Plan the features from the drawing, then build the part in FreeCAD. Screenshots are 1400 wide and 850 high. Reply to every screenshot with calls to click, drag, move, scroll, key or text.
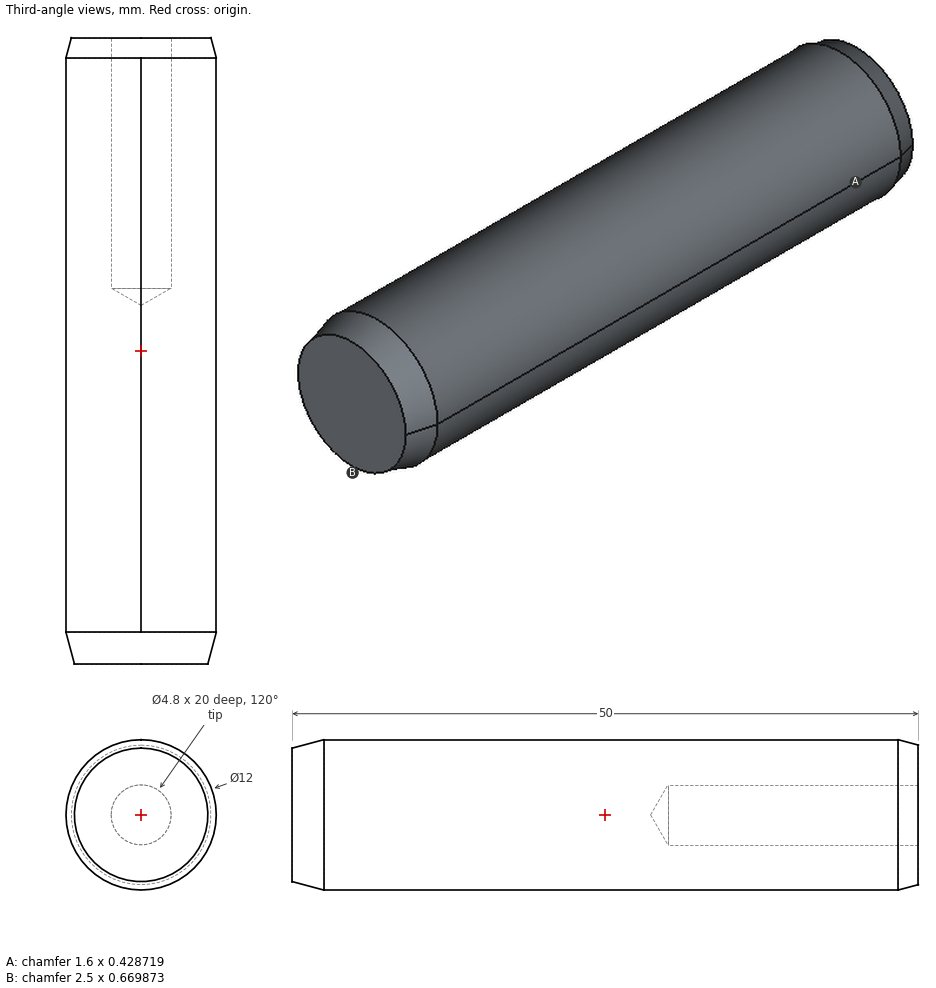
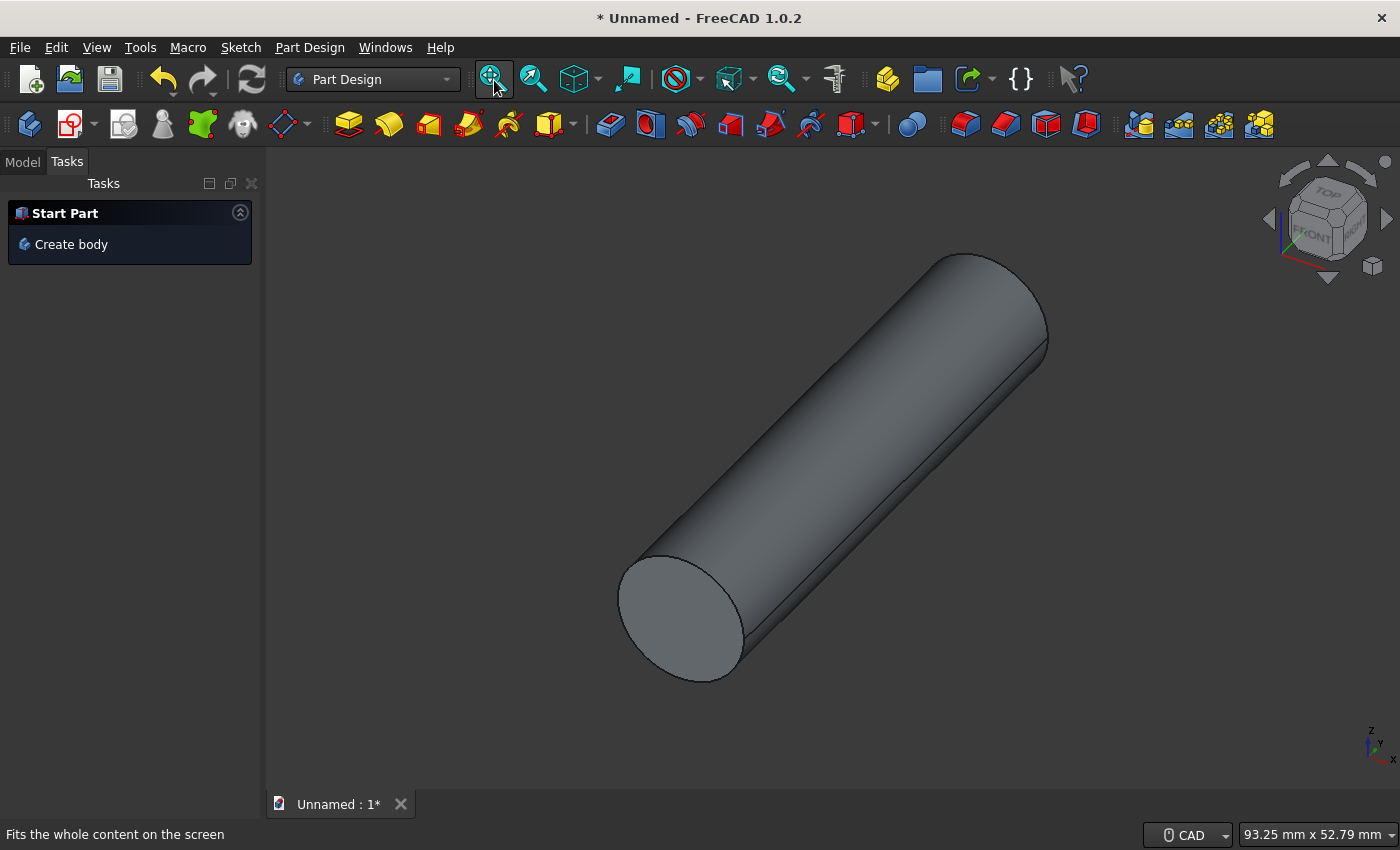
key(4)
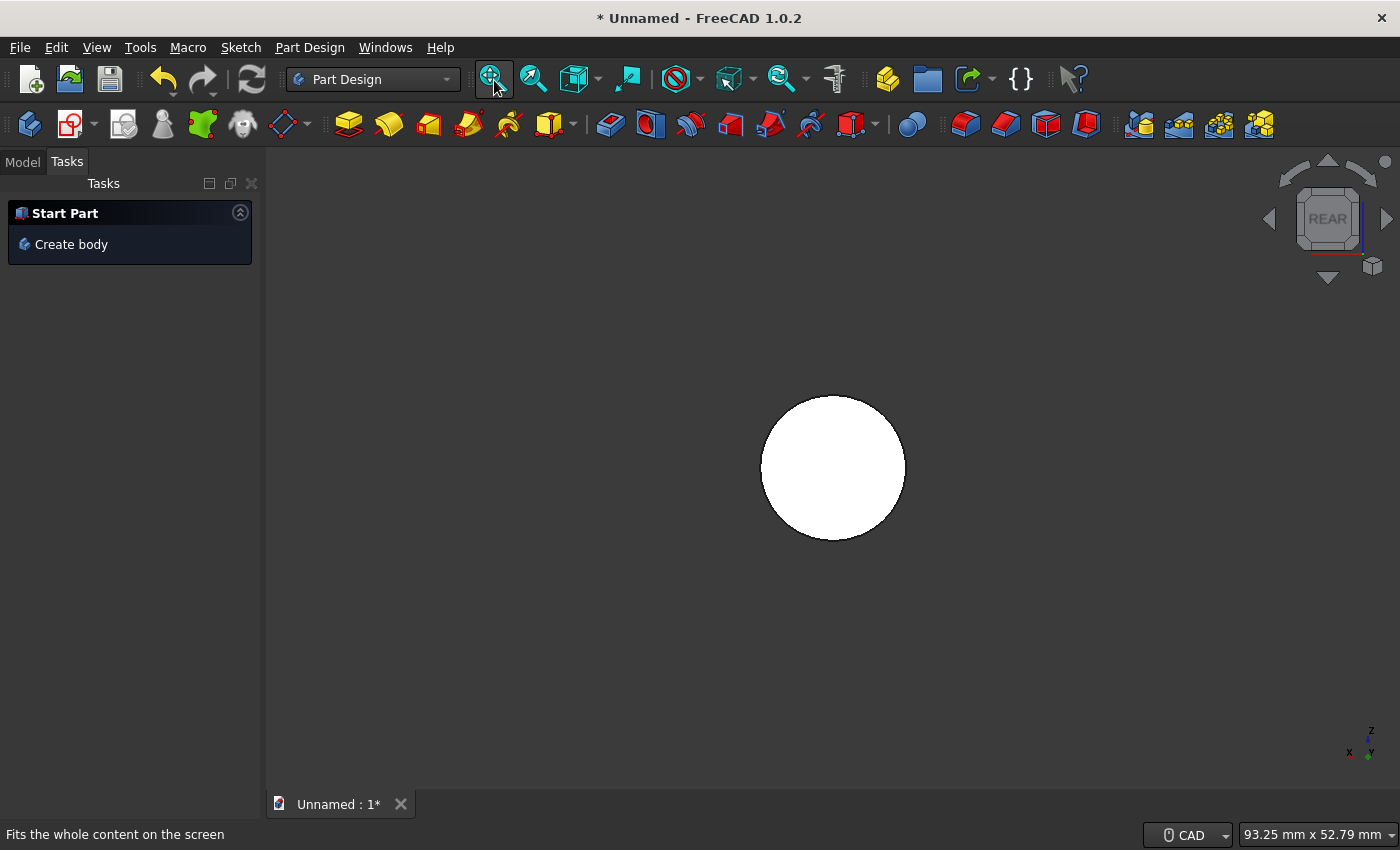
key(v)
key(f)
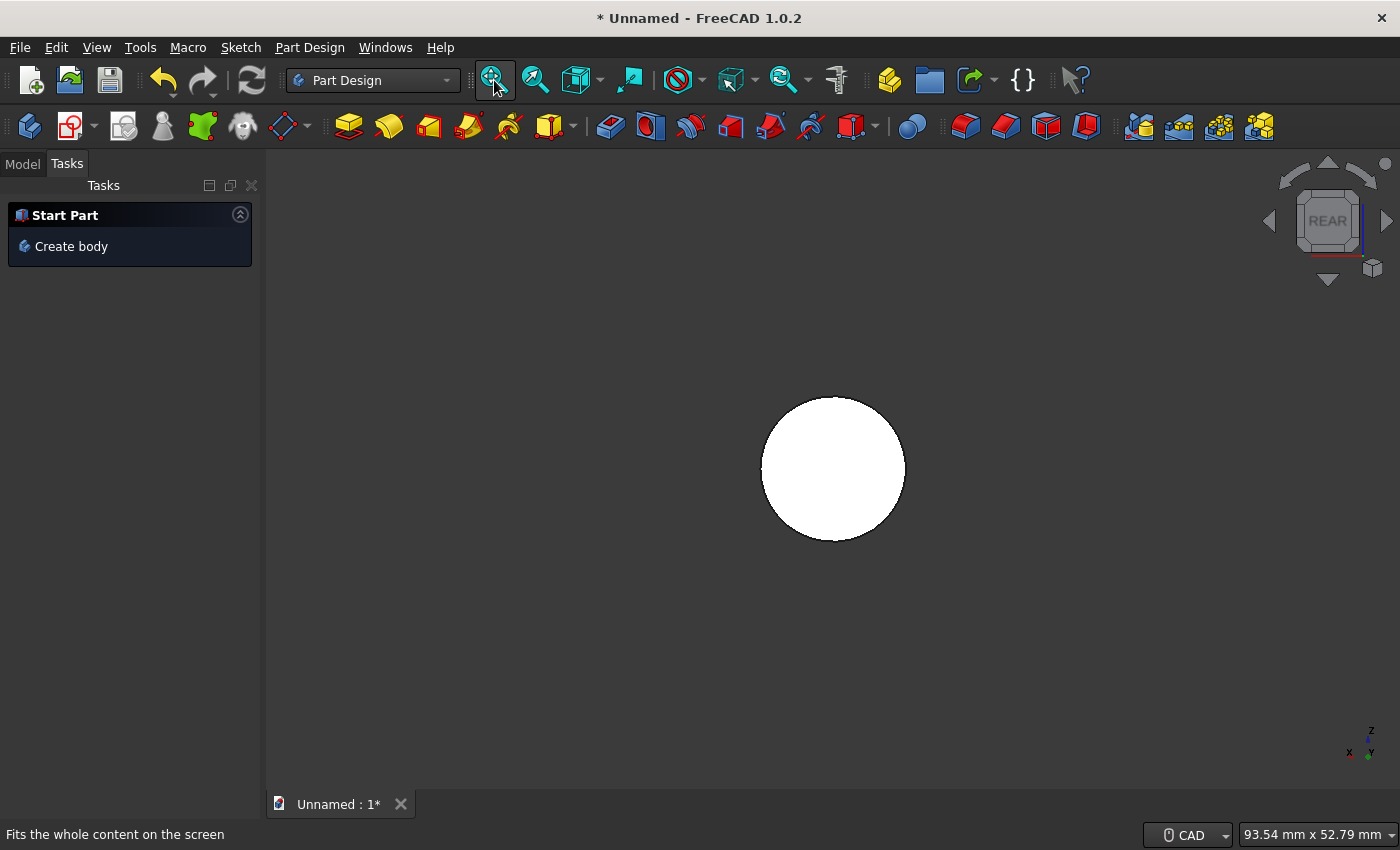
click(833, 468)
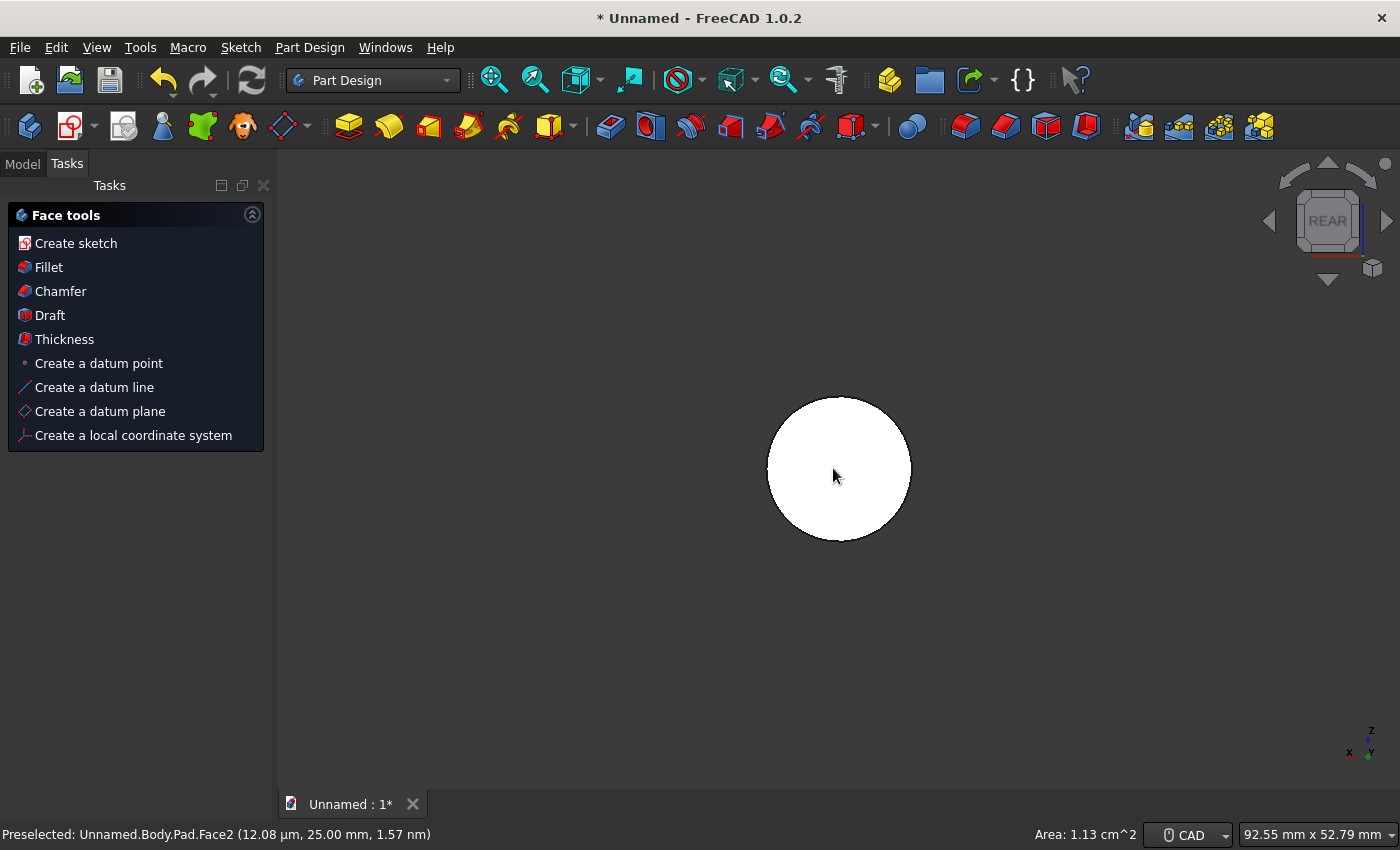
click(70, 126)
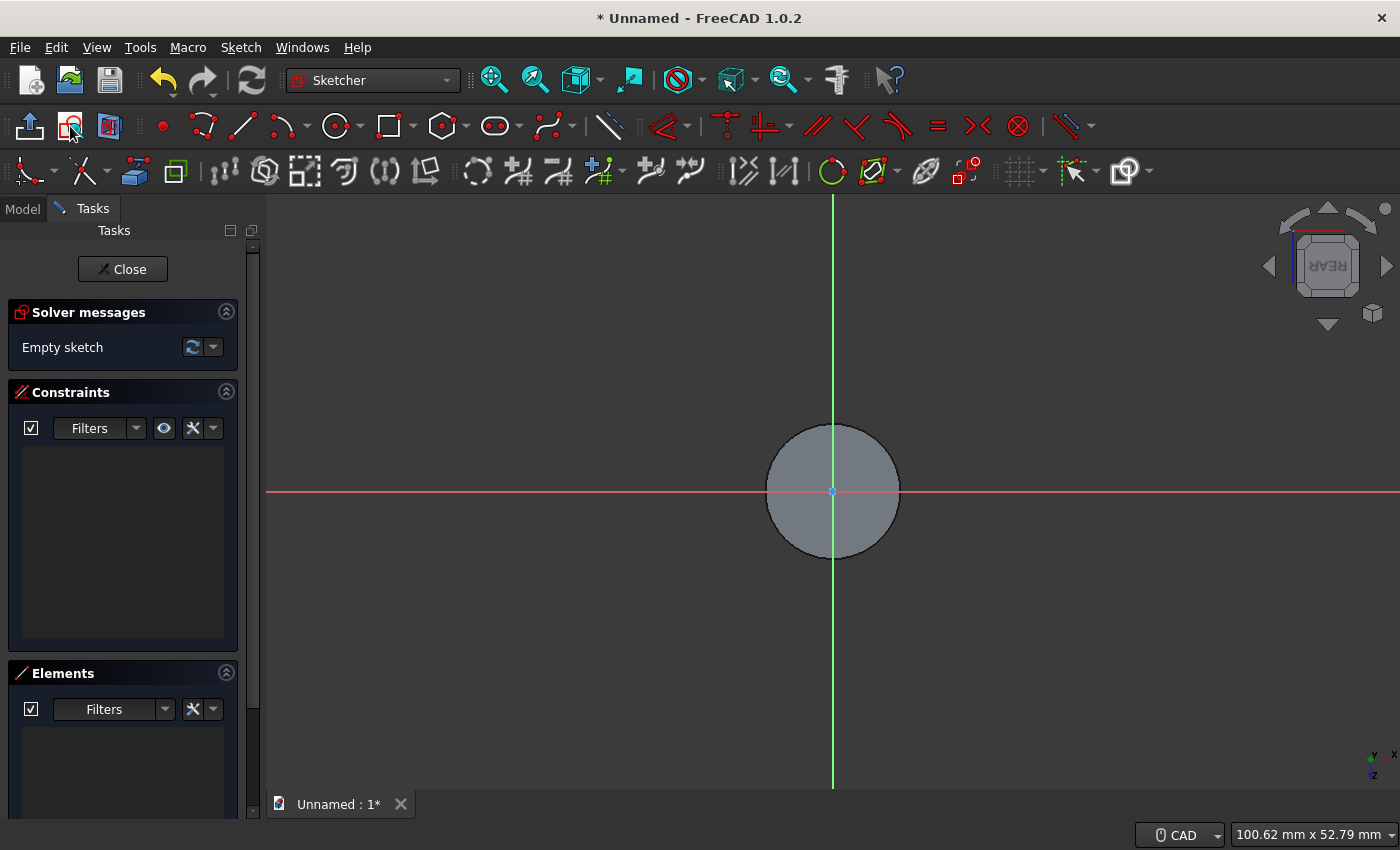
scroll(844, 491, up, 10)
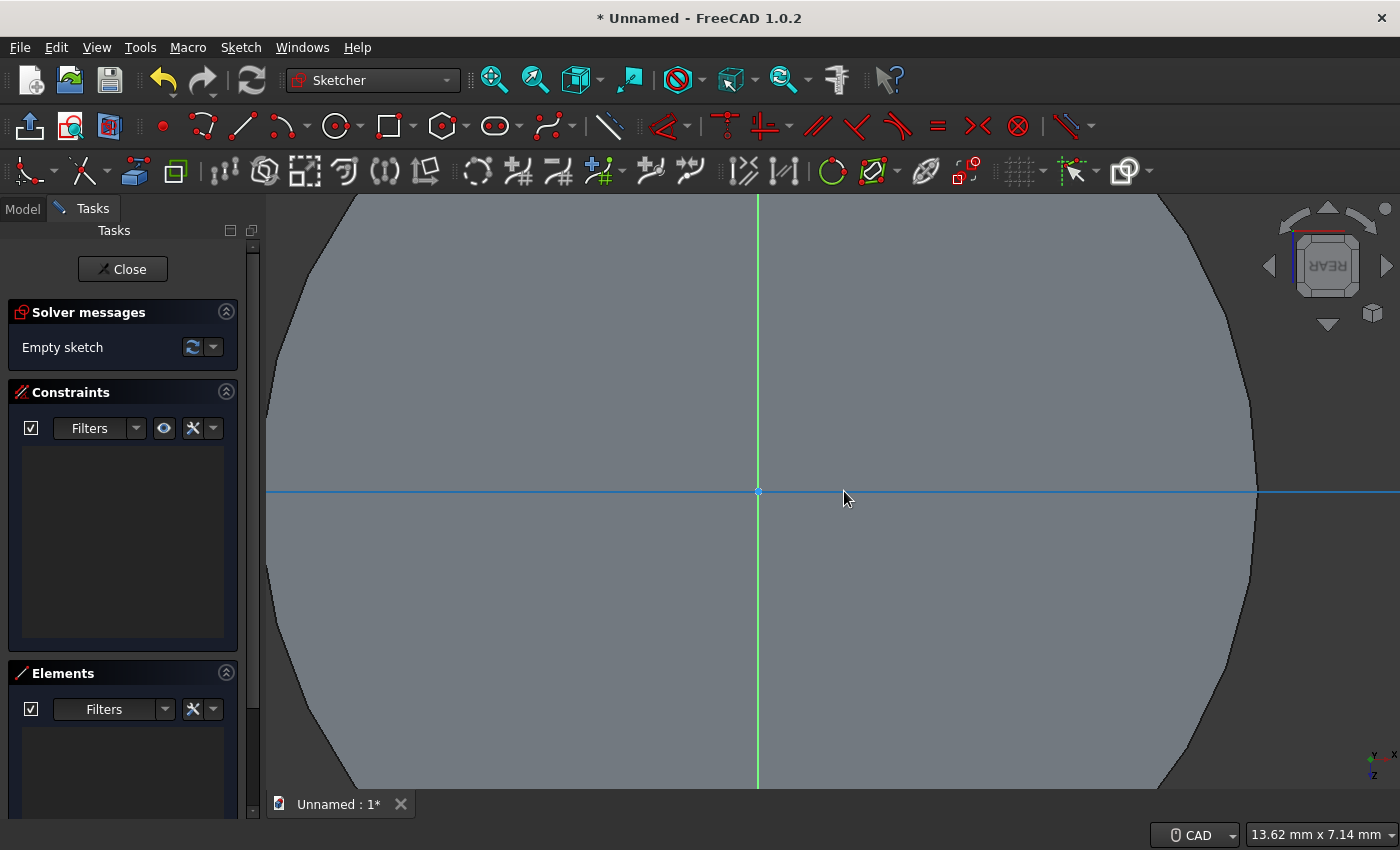
key(g)
key(c)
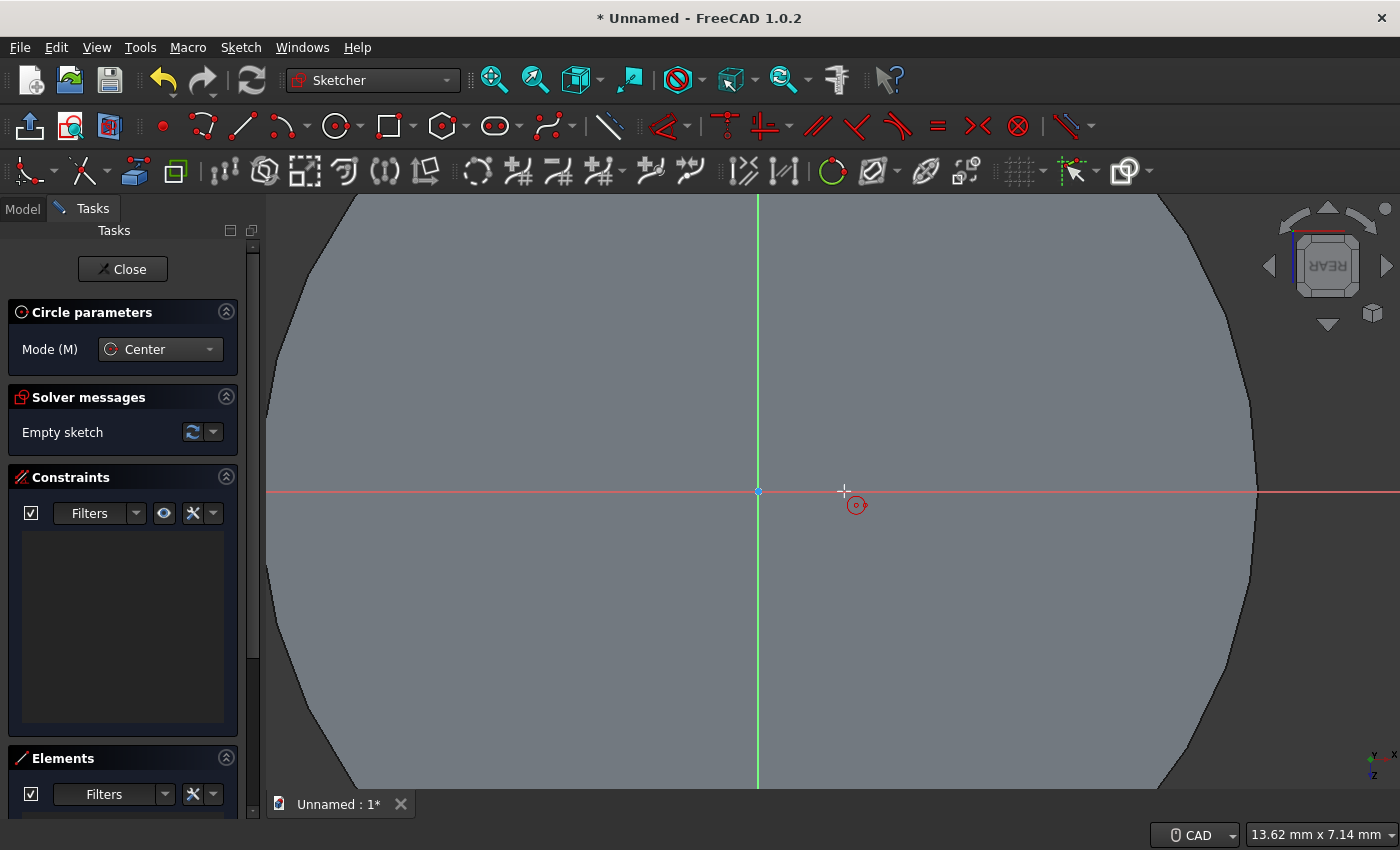
click(758, 491)
click(900, 350)
key(Escape)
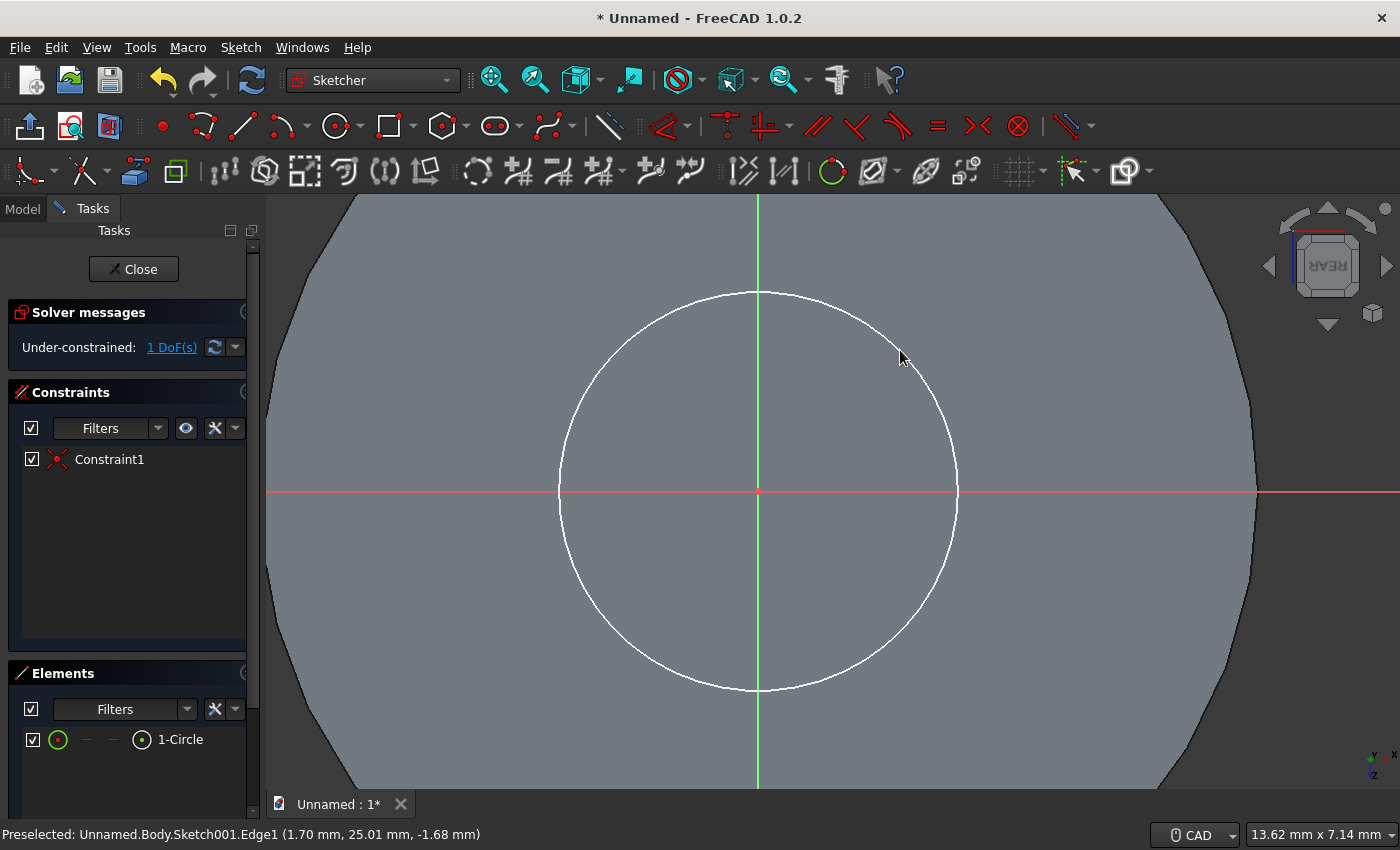
click(664, 126)